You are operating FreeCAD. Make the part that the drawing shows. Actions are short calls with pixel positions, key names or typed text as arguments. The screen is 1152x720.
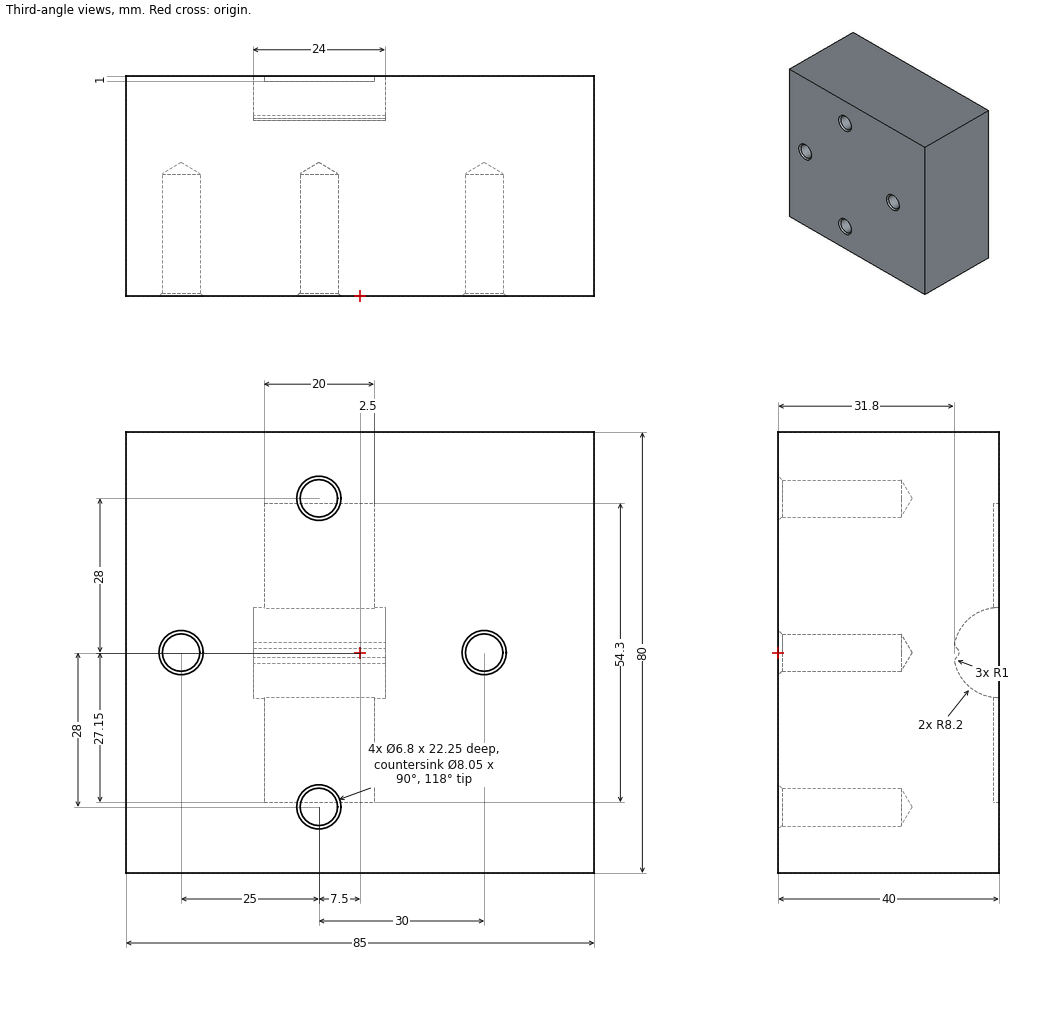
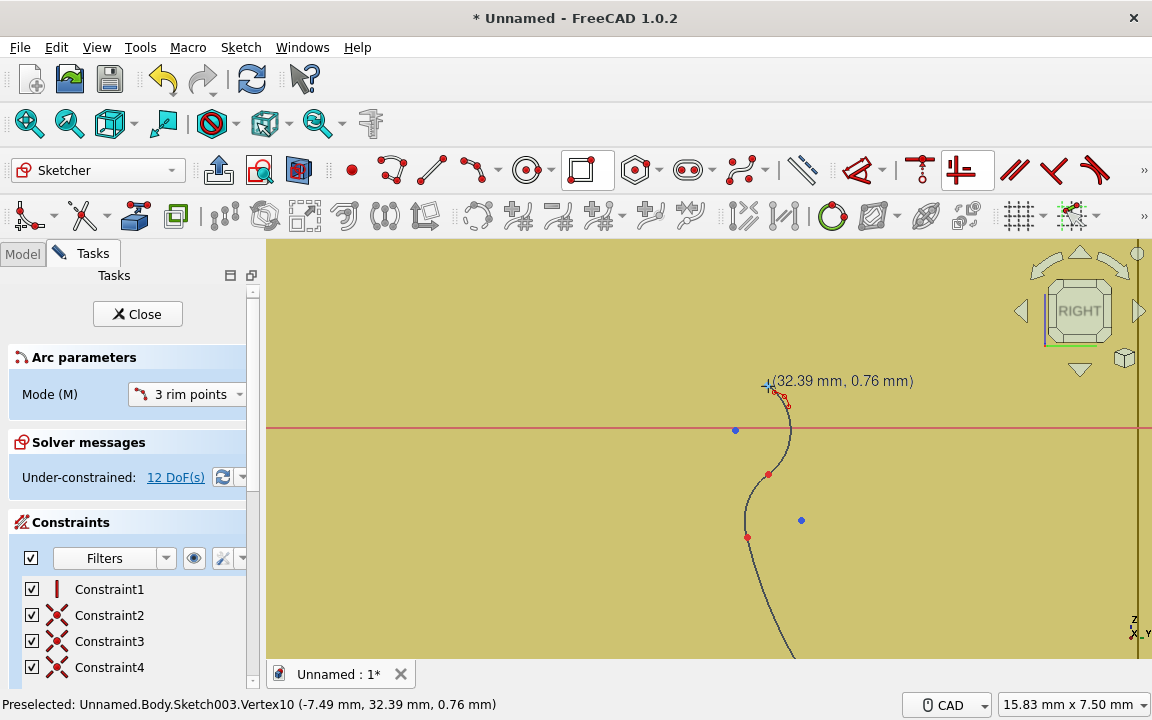
scroll(784, 454, down, 8)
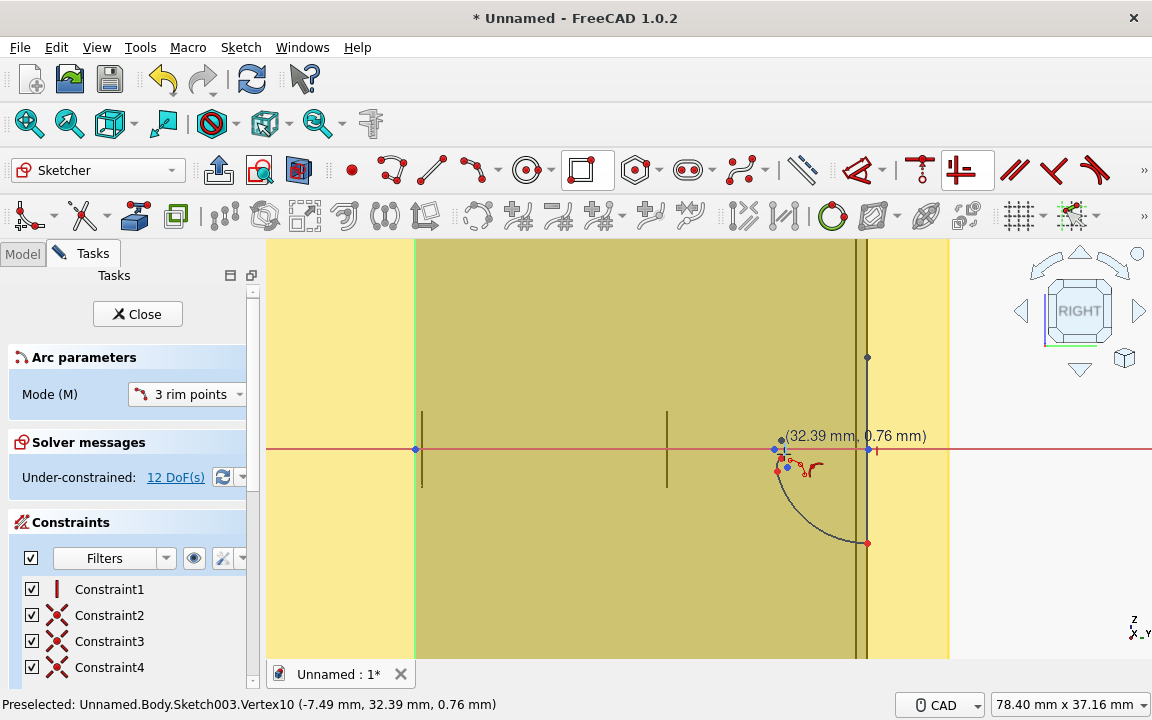
scroll(777, 428, up, 2)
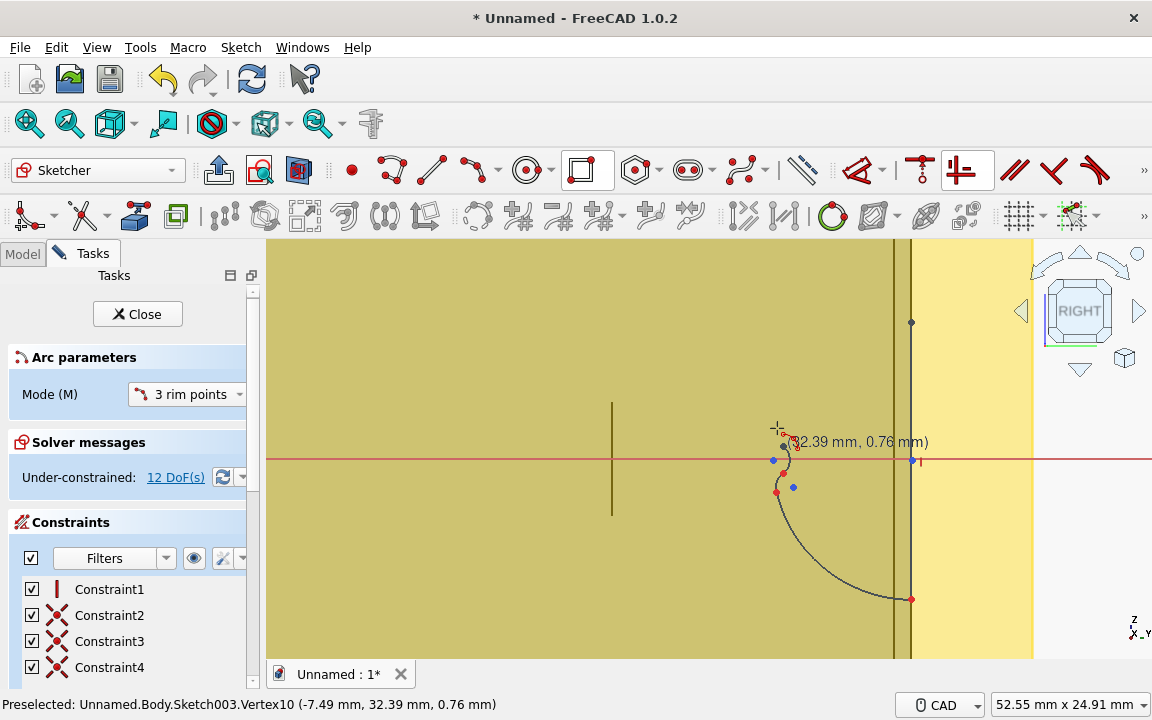
click(777, 428)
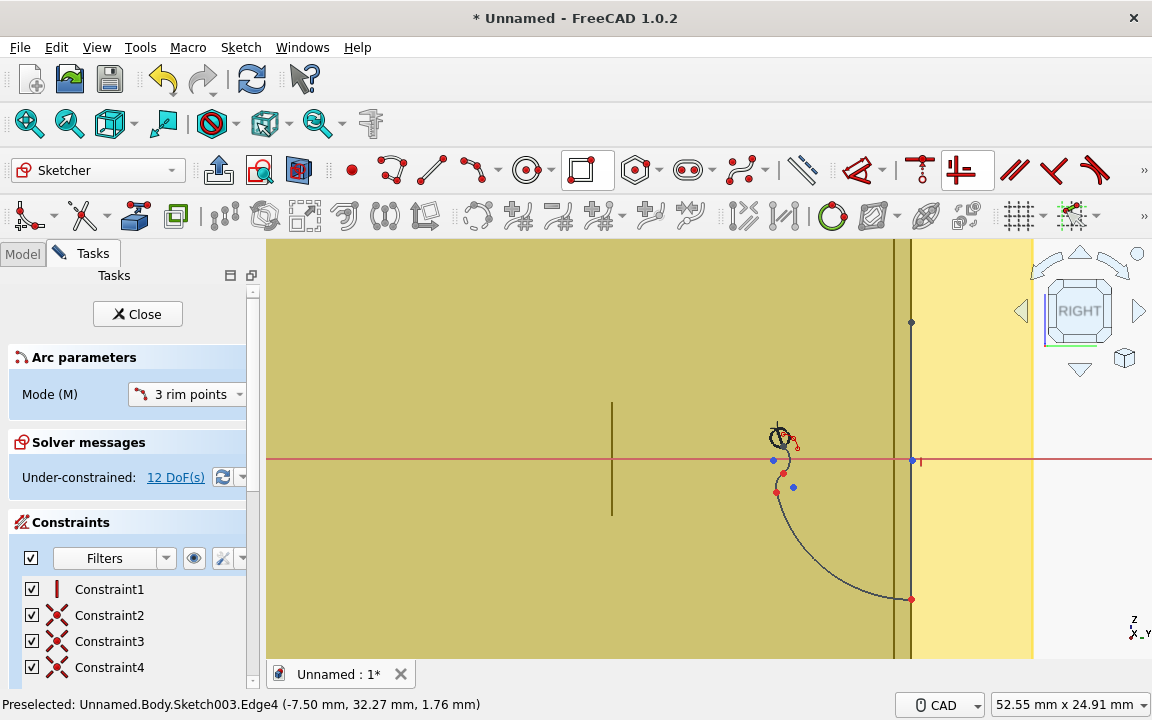
scroll(777, 438, up, 9)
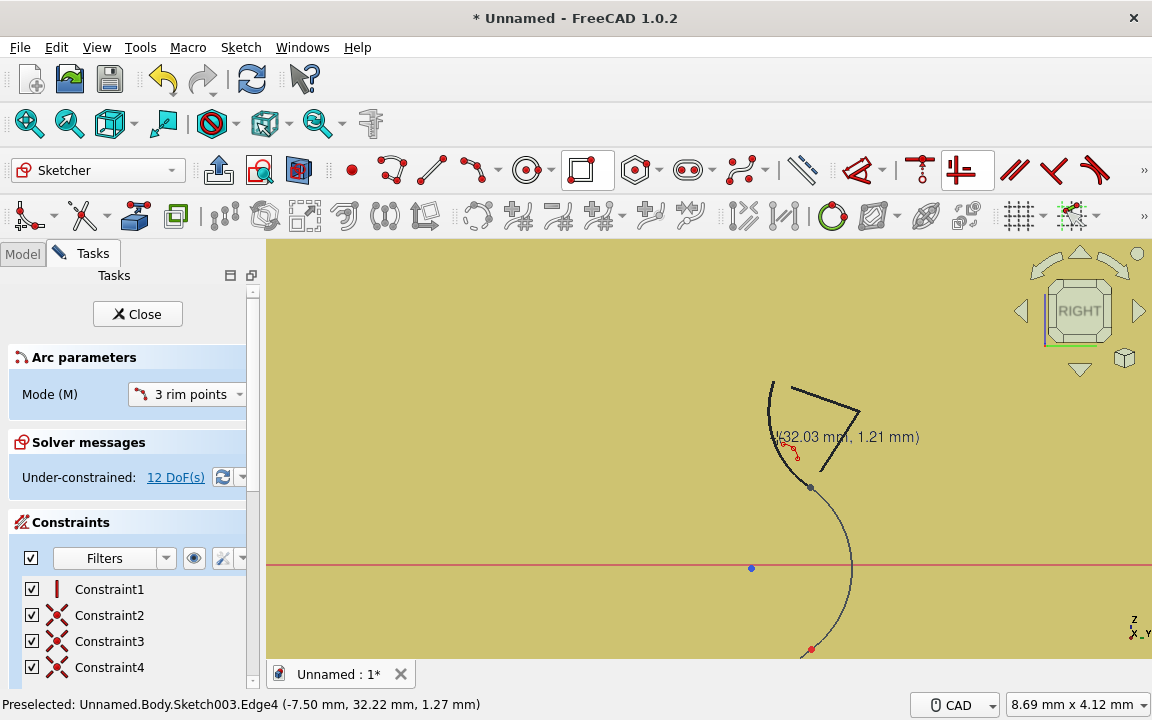
click(775, 436)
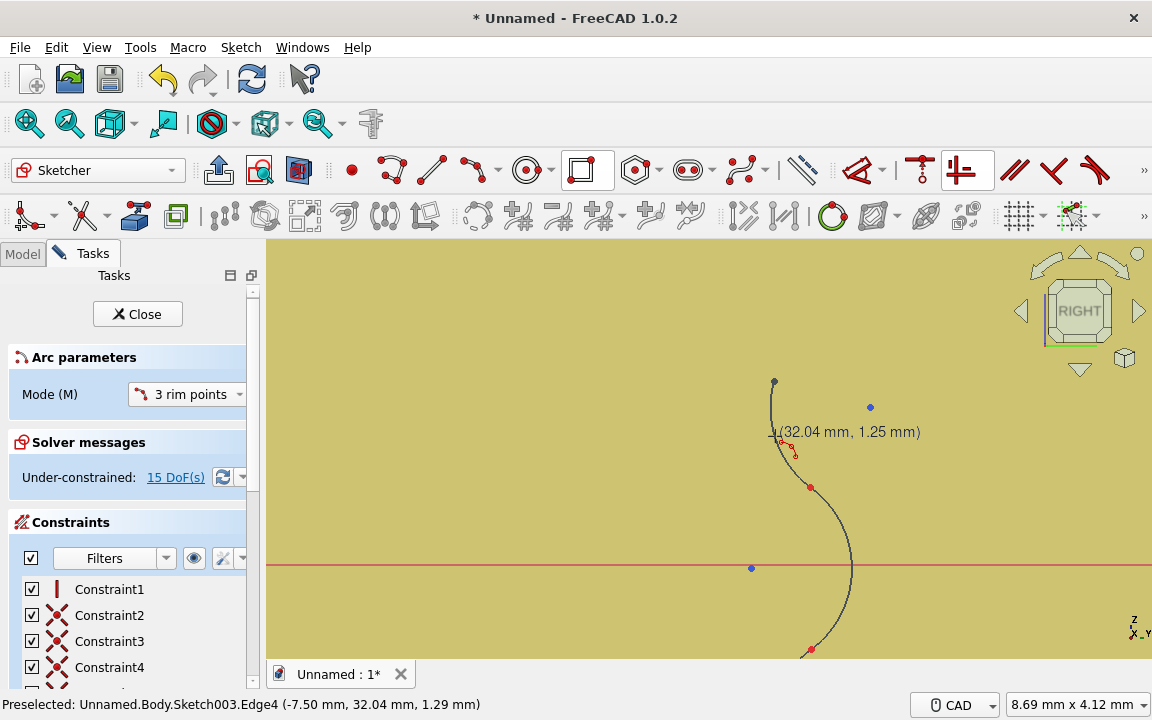
scroll(777, 435, down, 11)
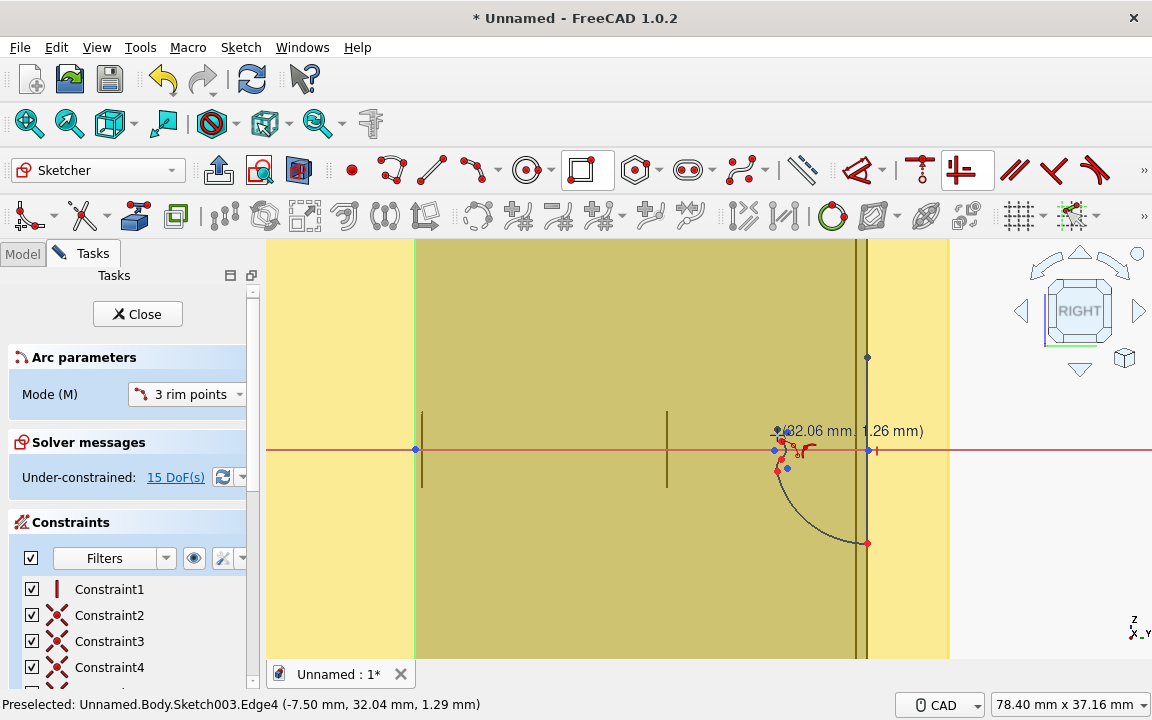
scroll(777, 429, up, 2)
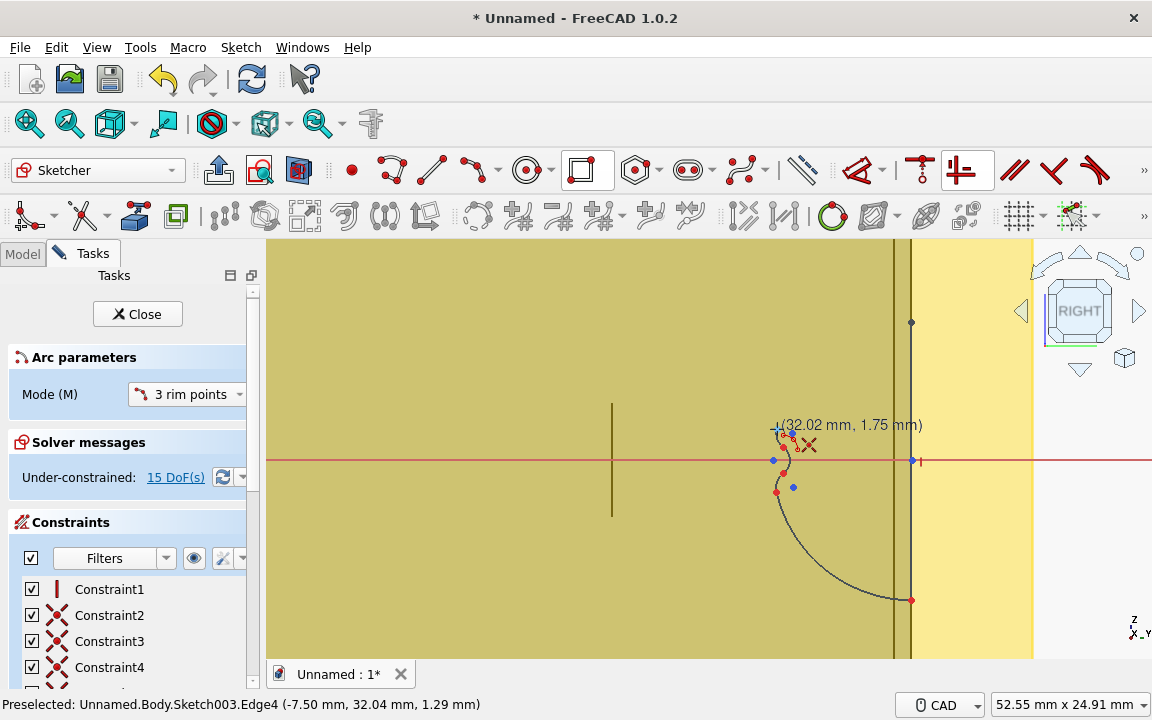
click(777, 429)
click(911, 323)
click(825, 352)
key(Escape)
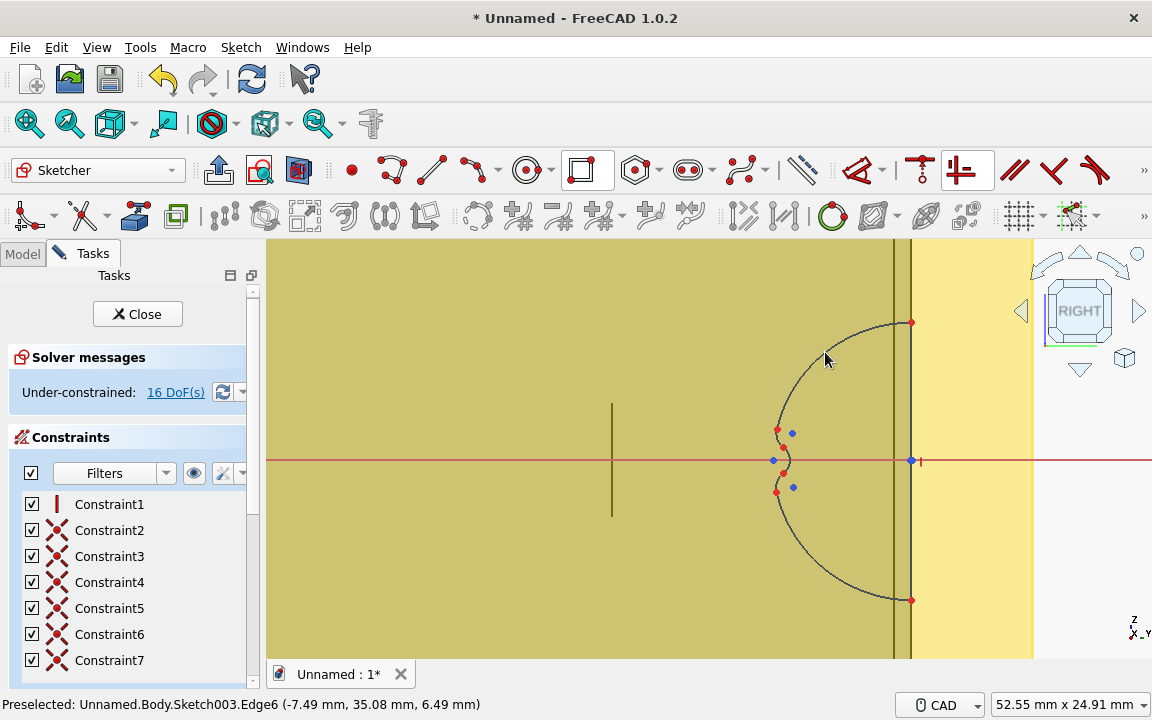
click(800, 543)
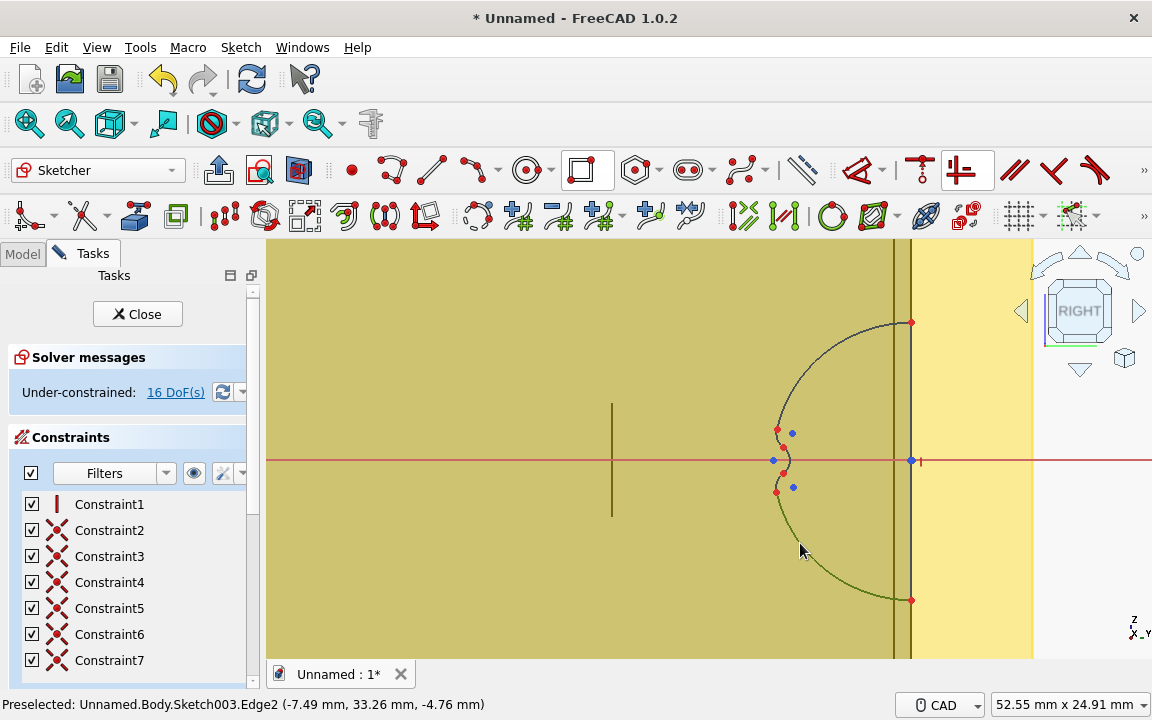
scroll(777, 482, up, 2)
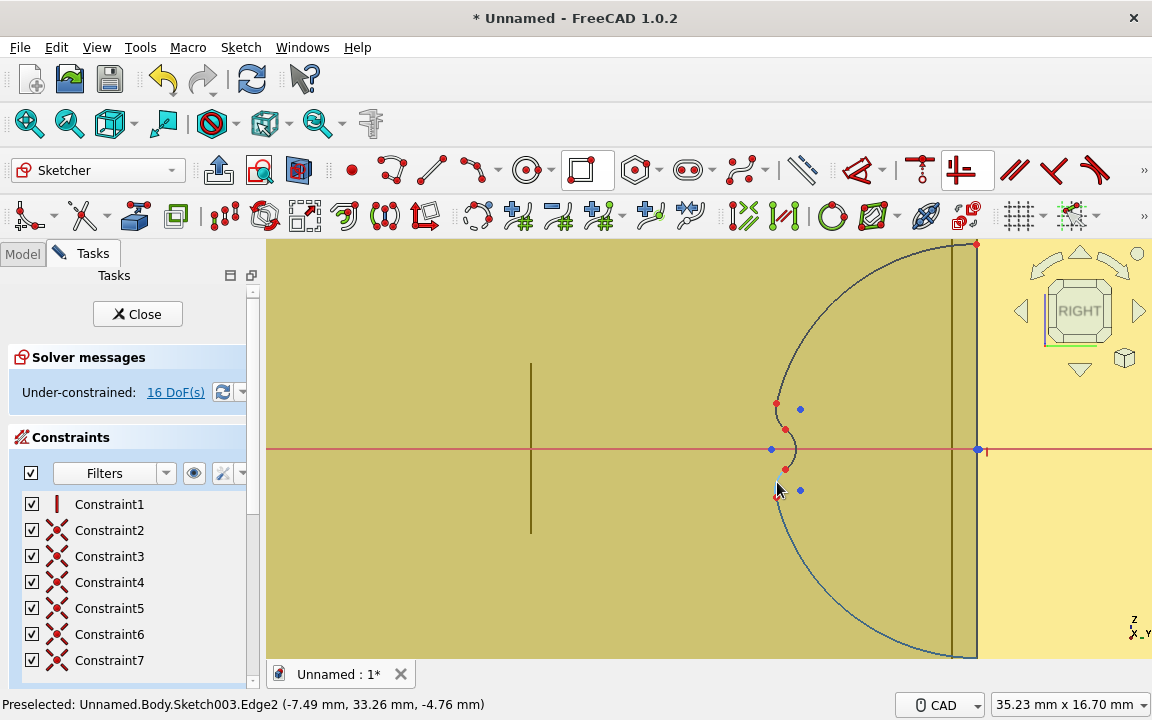
click(777, 482)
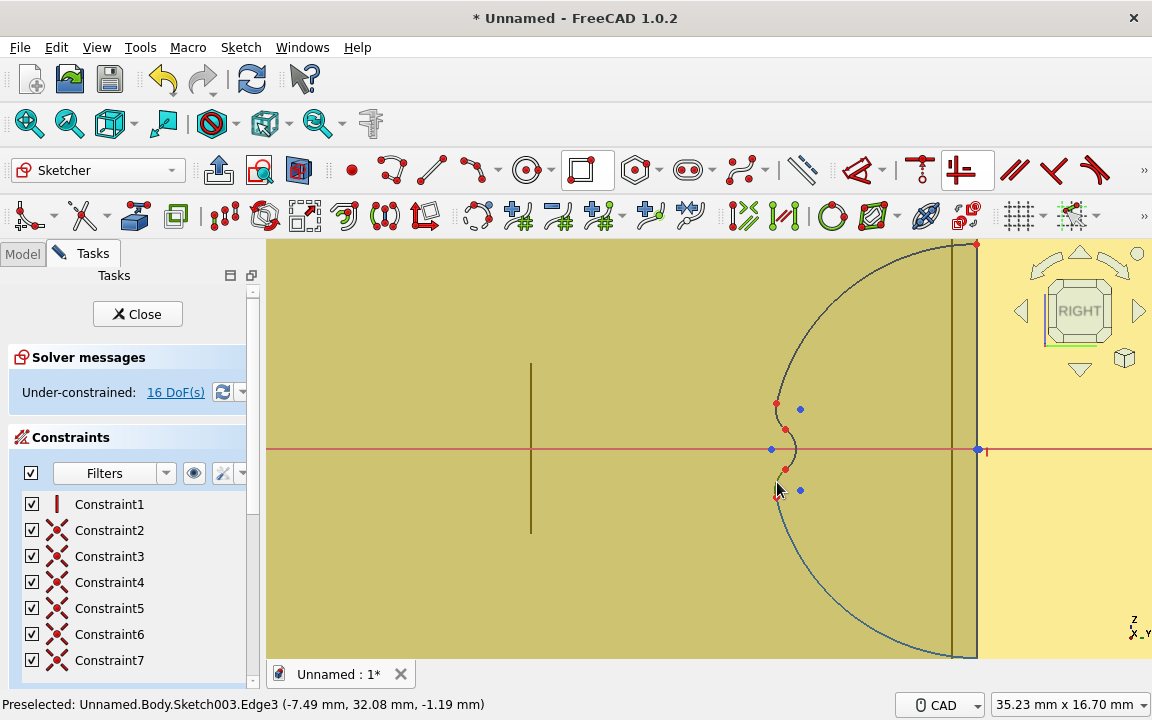
click(1096, 170)